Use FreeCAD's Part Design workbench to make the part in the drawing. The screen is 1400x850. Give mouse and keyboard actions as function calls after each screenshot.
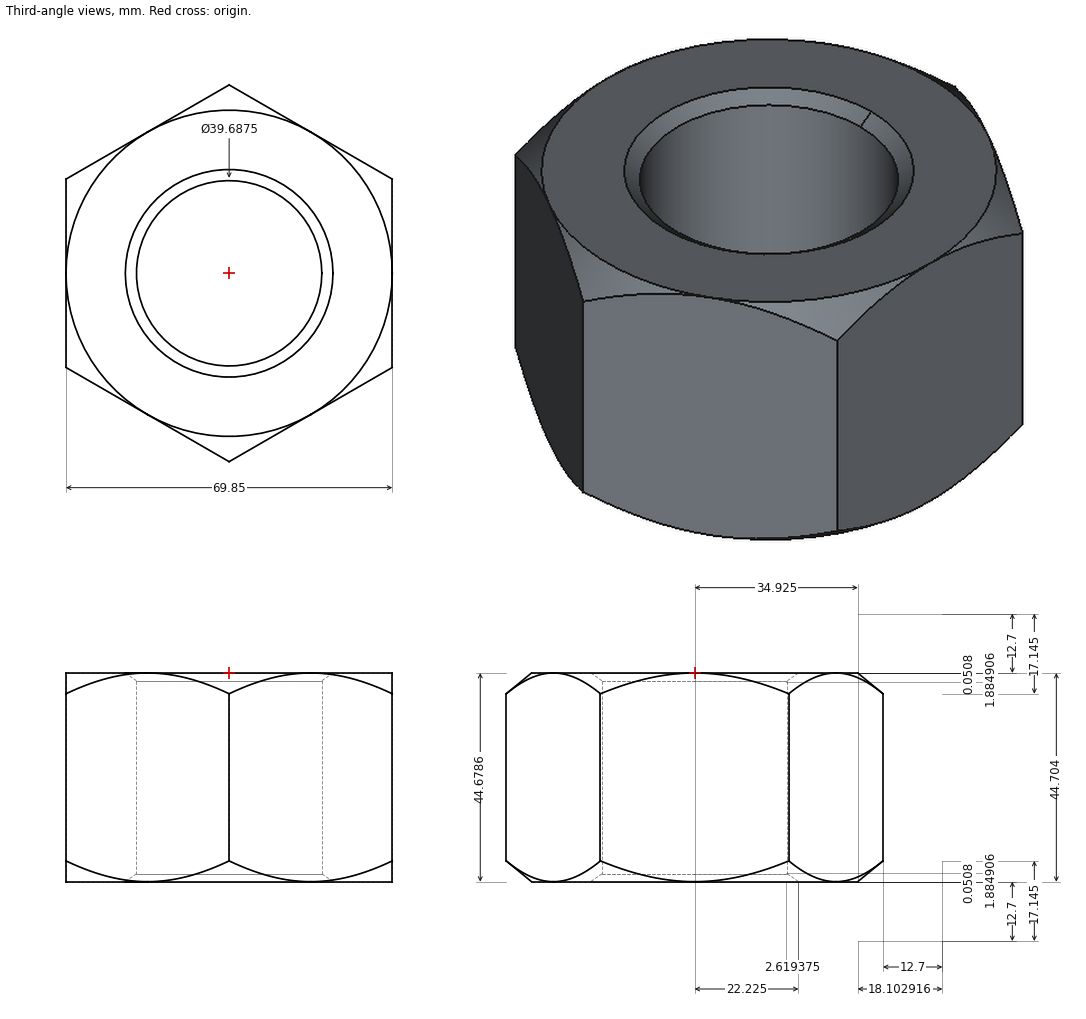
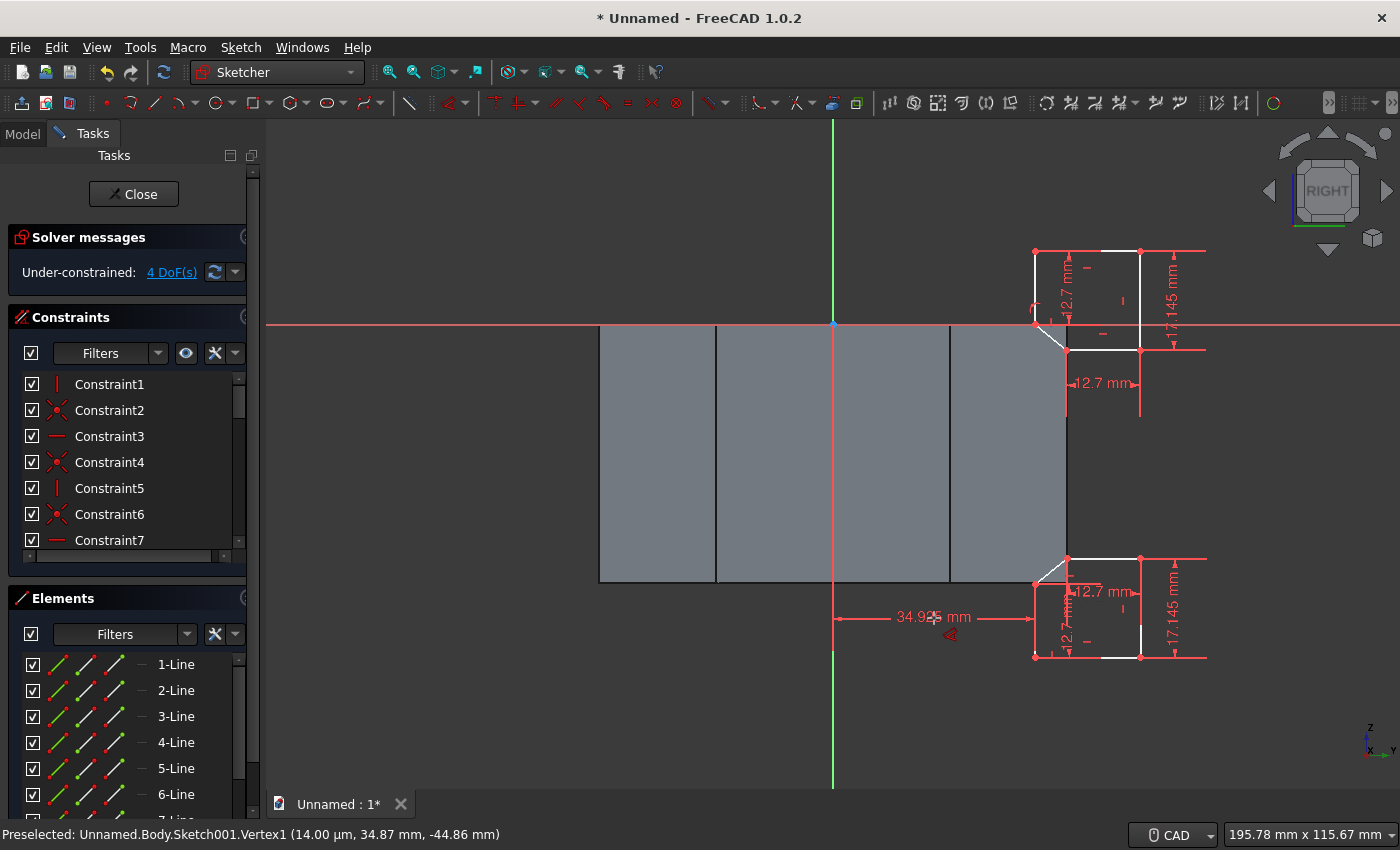
click(1035, 325)
click(934, 291)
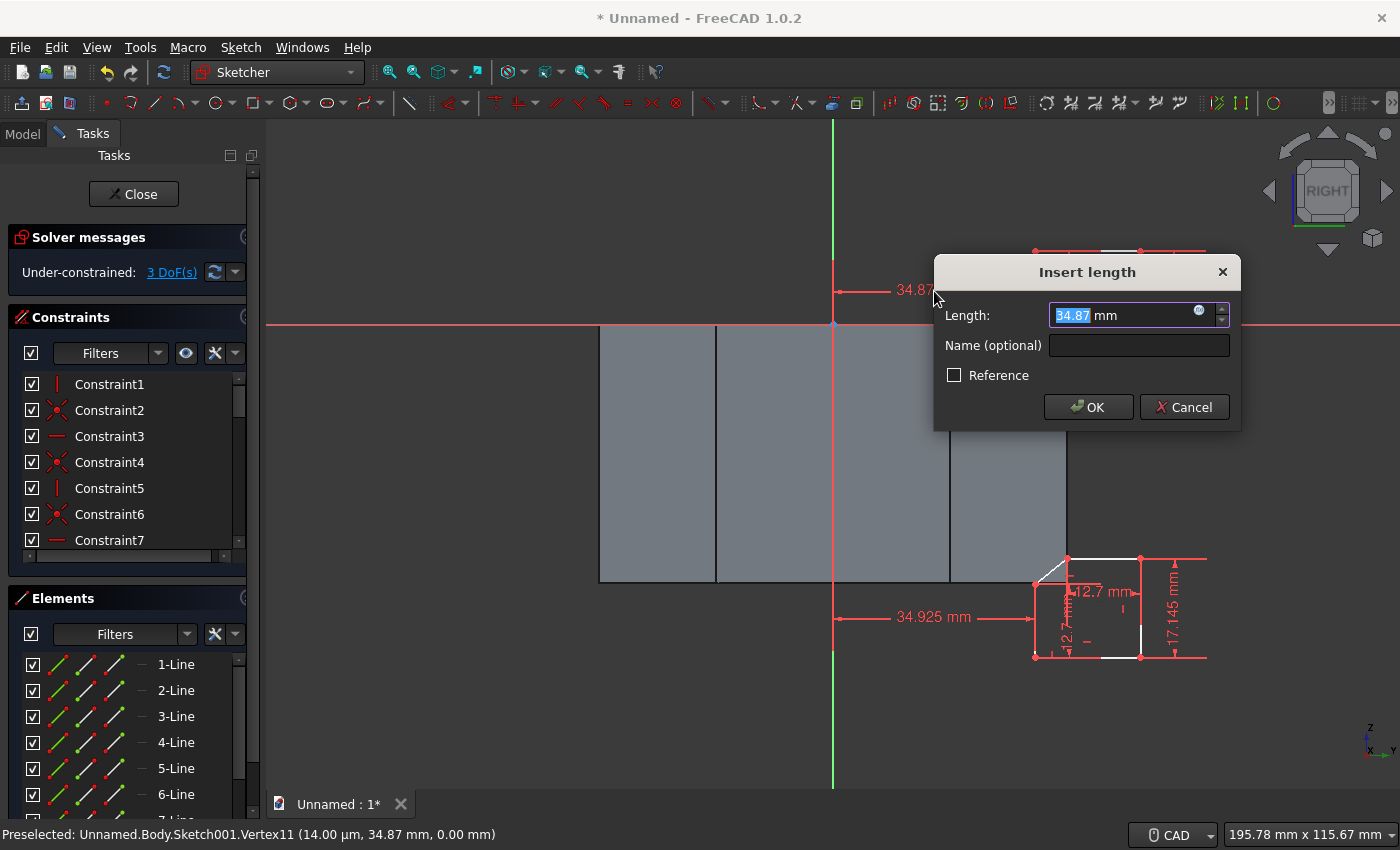
text(34.925)
key(Return)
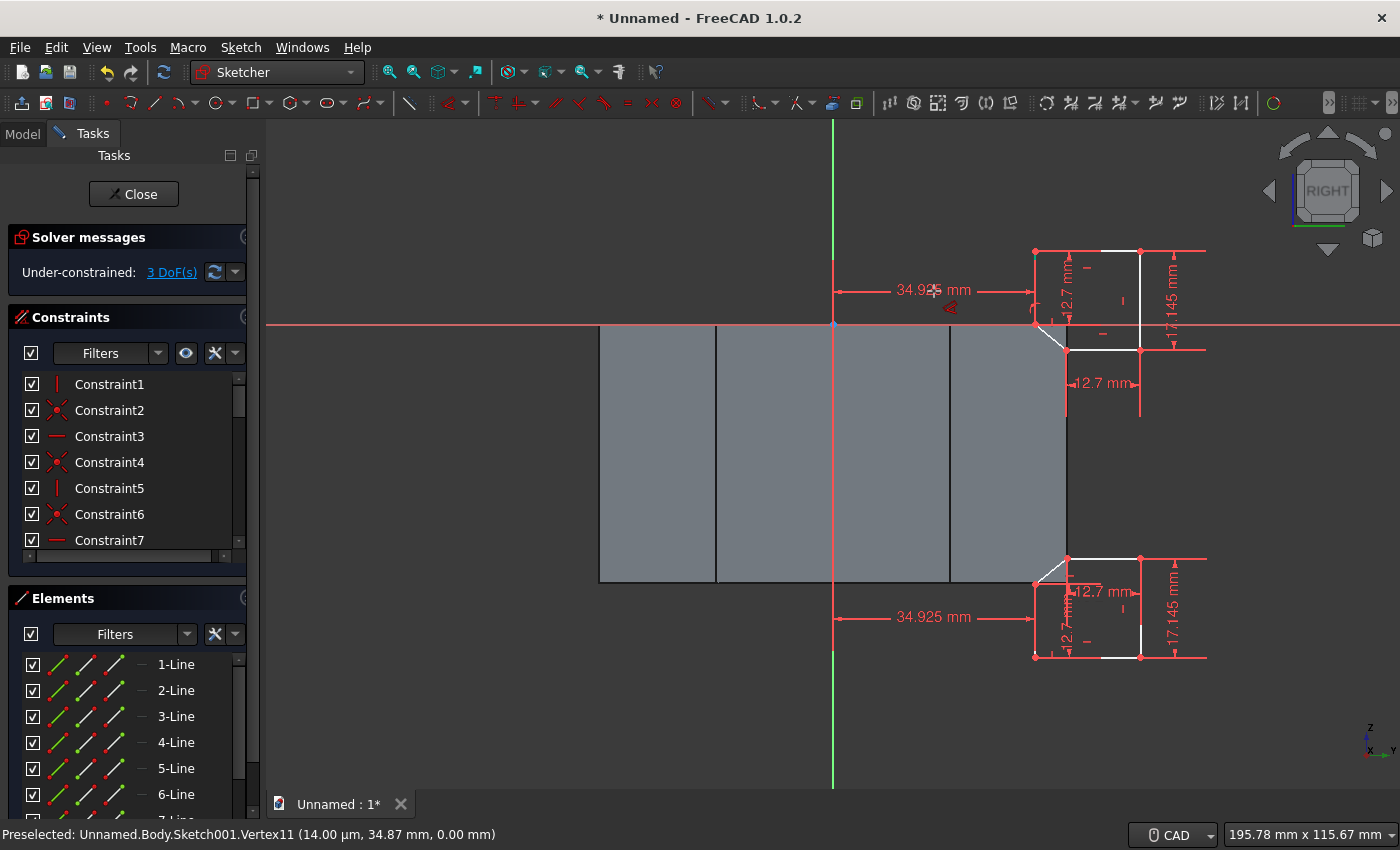
click(1035, 584)
click(799, 455)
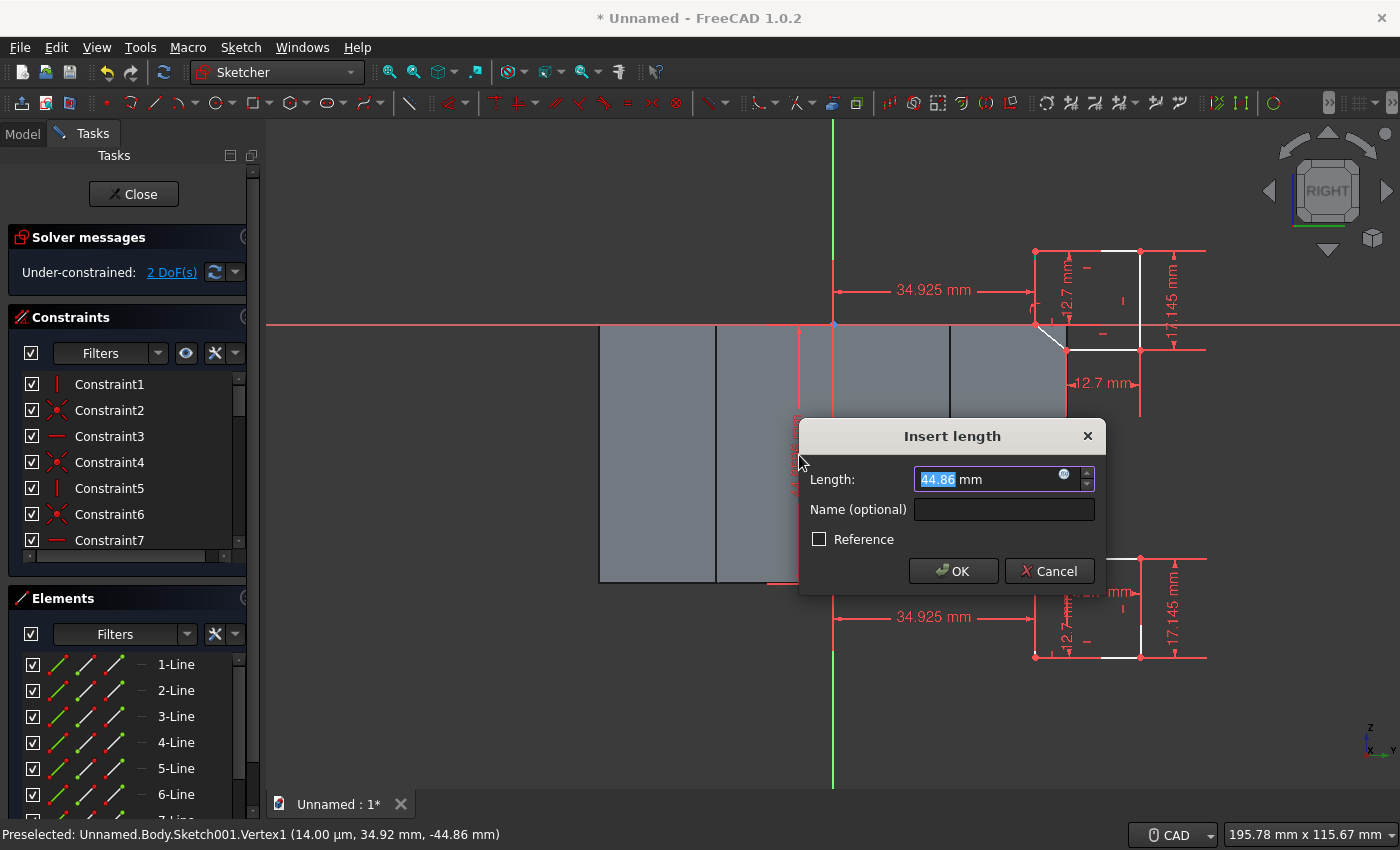
text(44.6786)
key(Return)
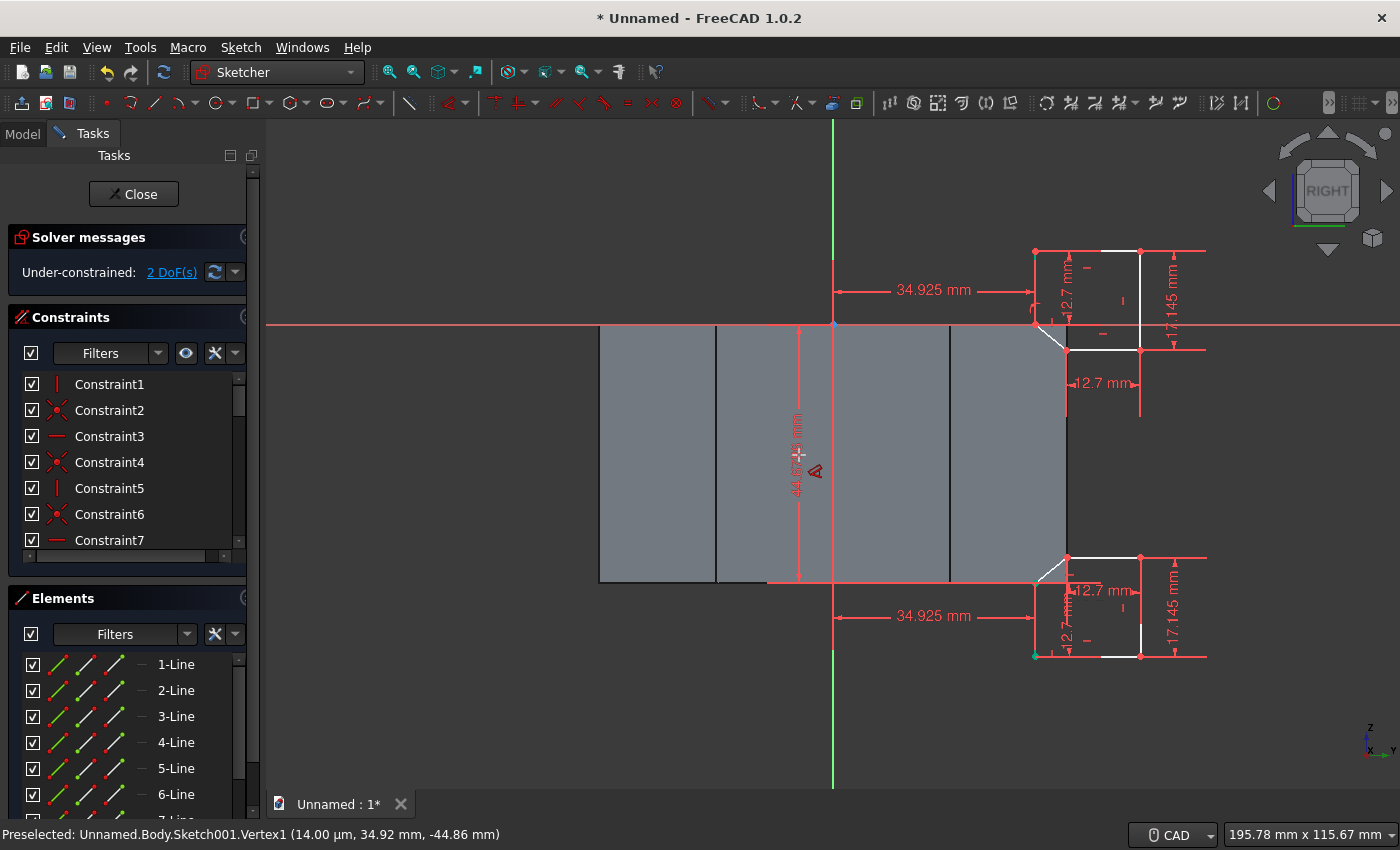
click(1067, 657)
click(1088, 691)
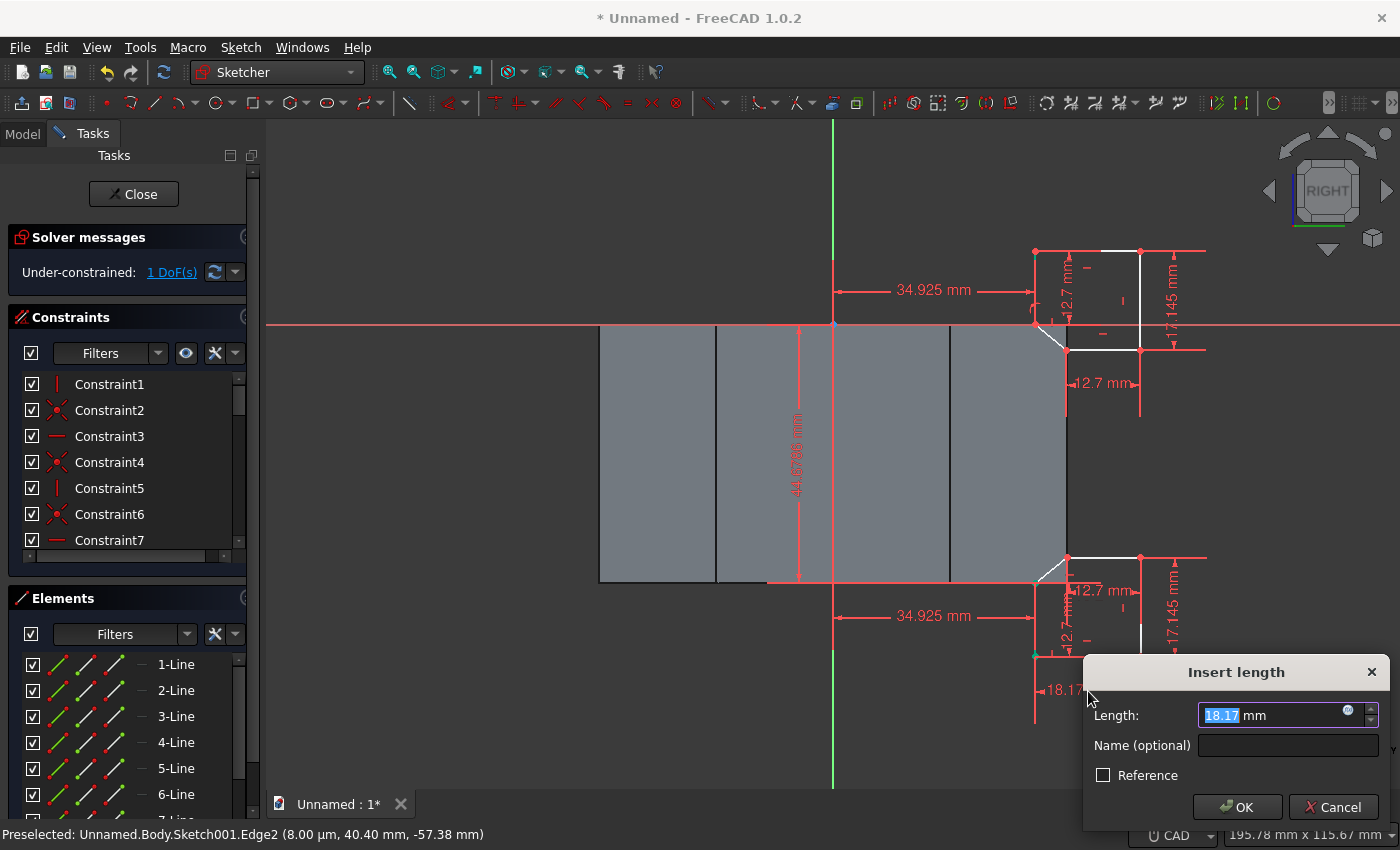
text(18.102916)
key(Return)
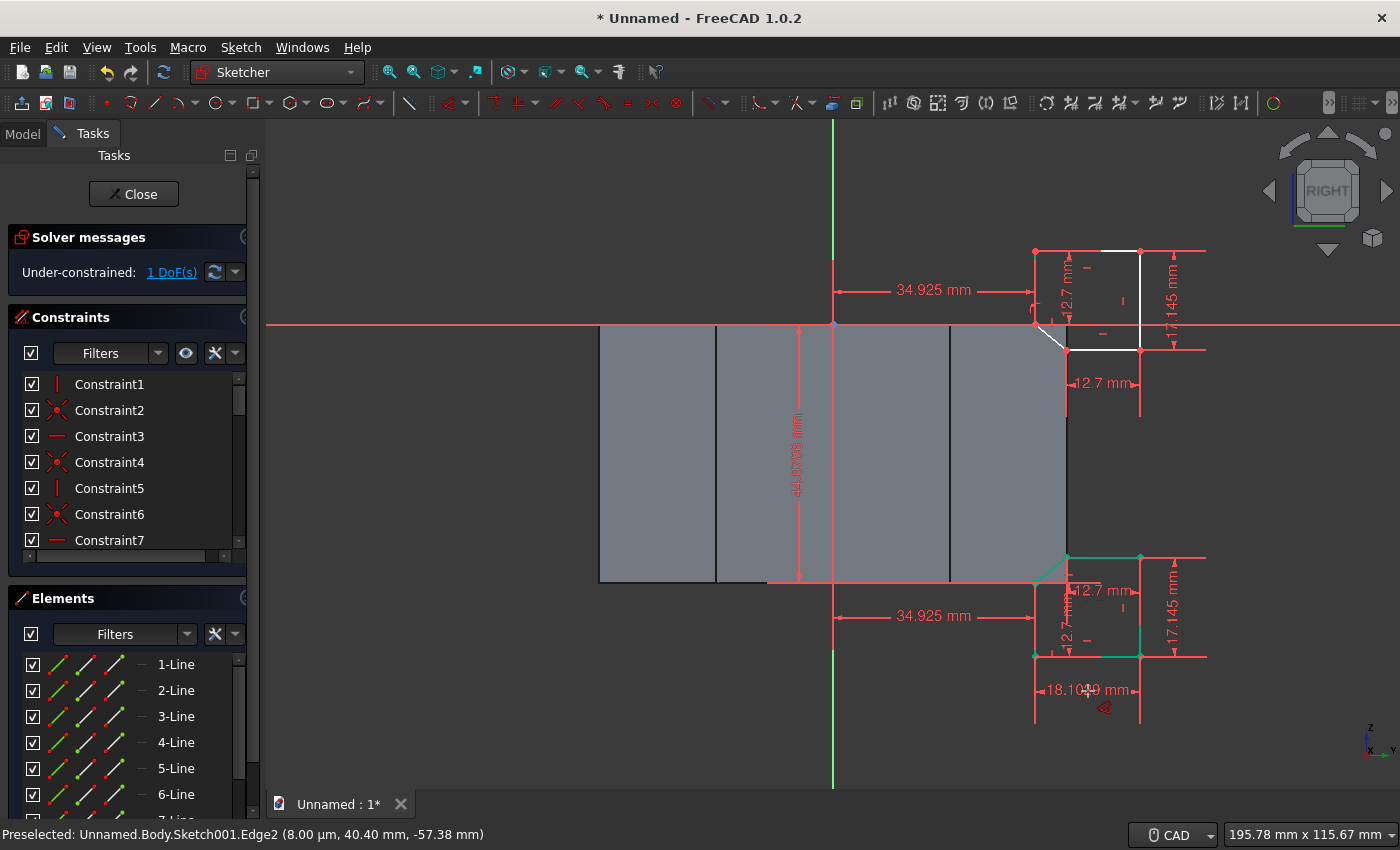
click(1109, 251)
click(1088, 217)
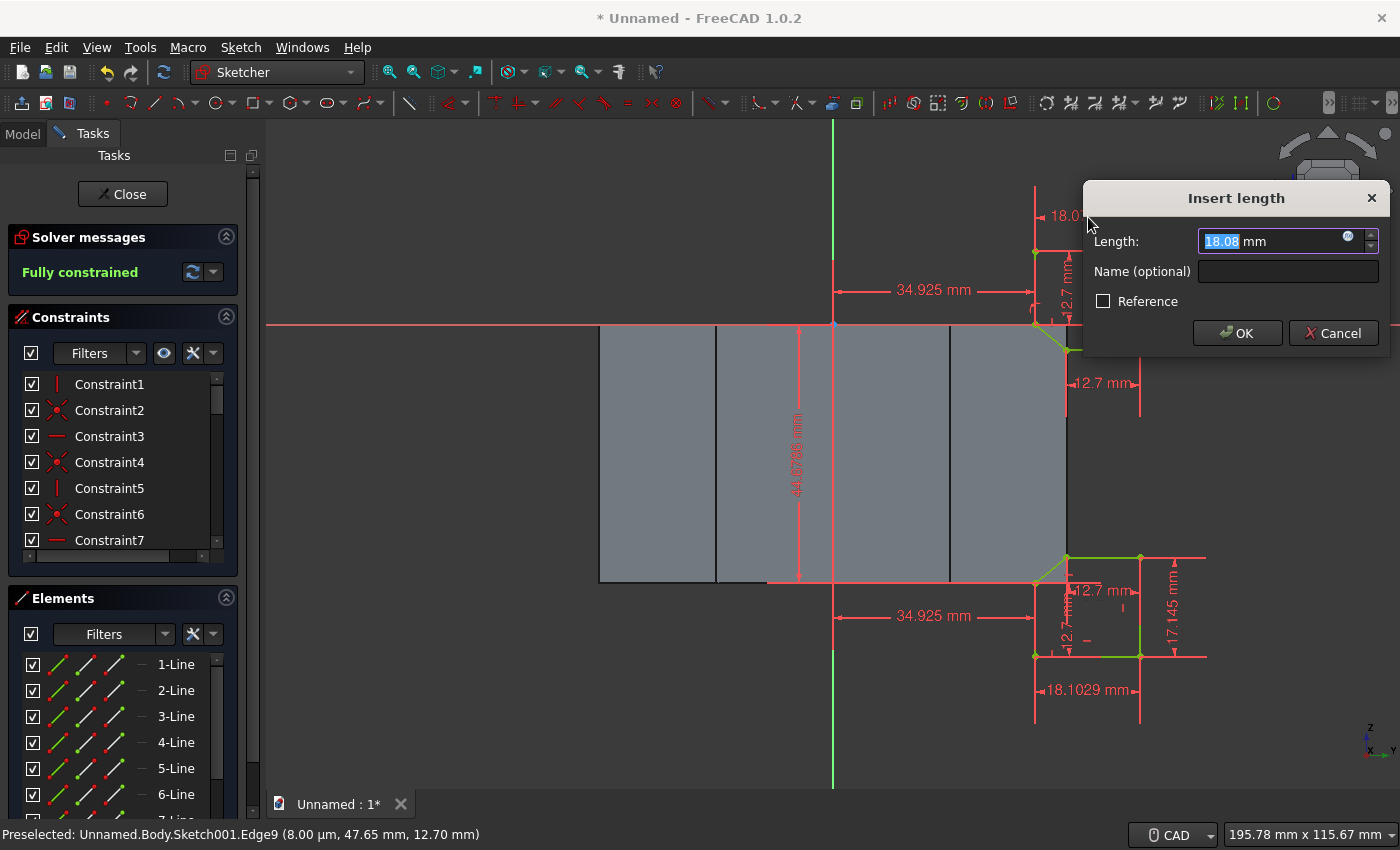
text(18.102916)
key(Return)
key(Escape)